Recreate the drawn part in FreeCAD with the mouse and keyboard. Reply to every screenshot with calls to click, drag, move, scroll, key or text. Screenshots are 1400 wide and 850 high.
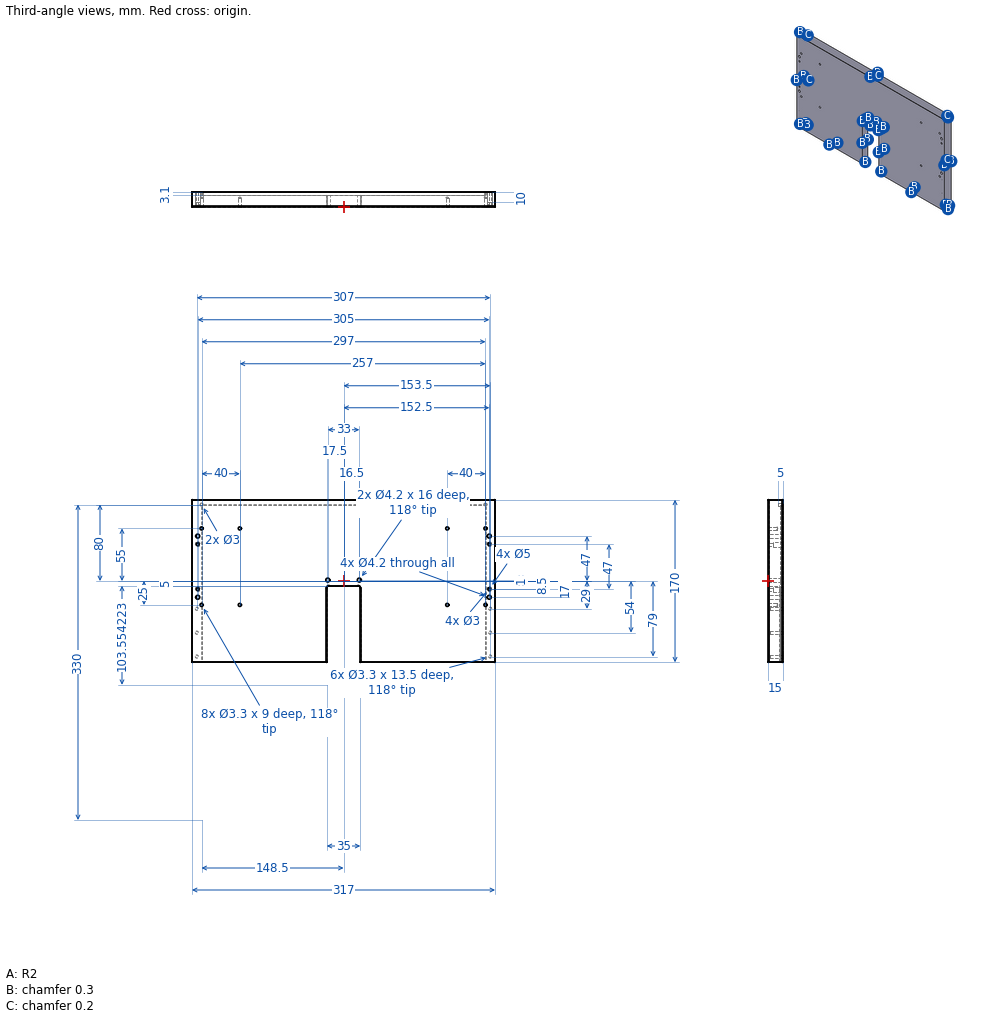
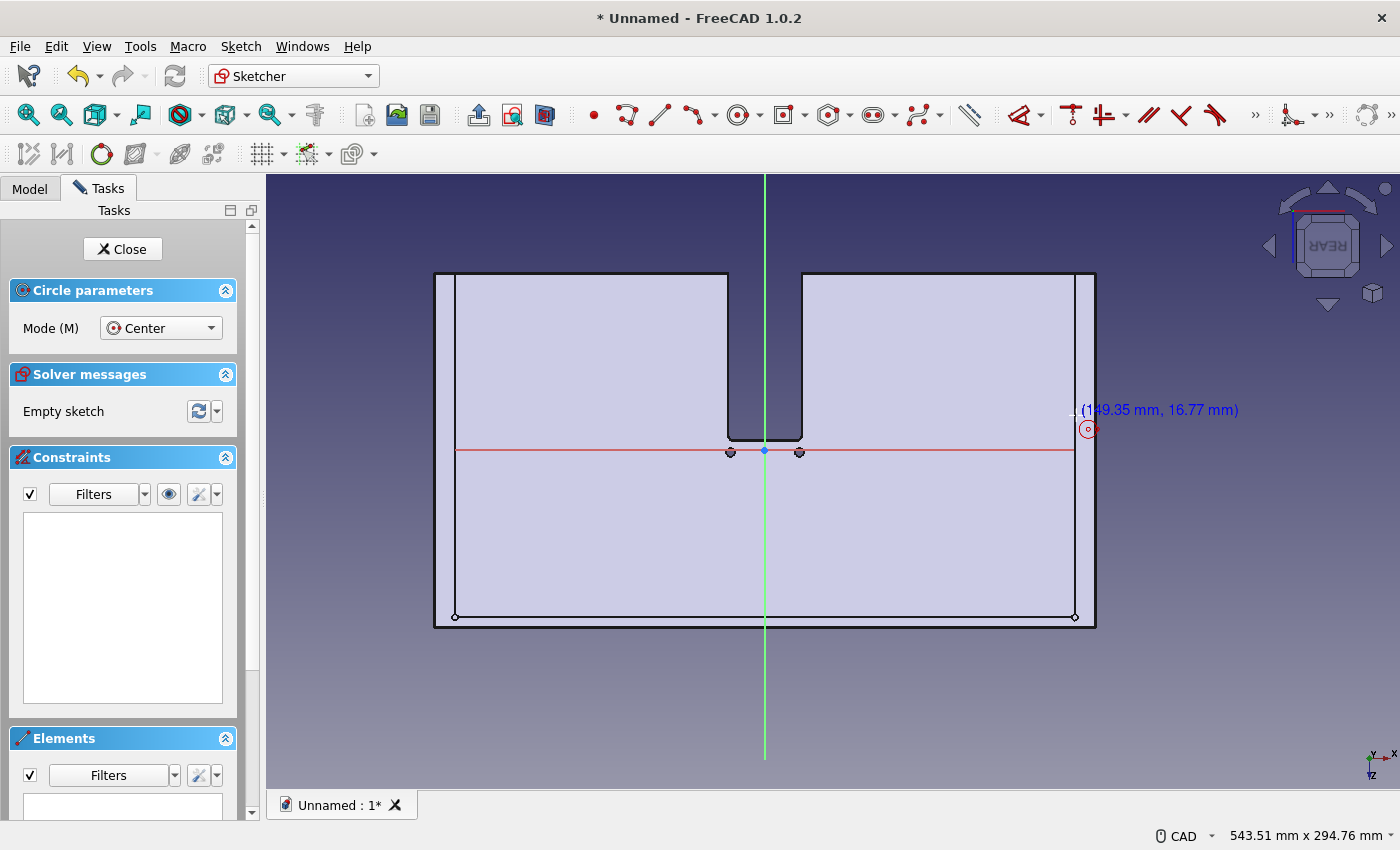
click(1083, 415)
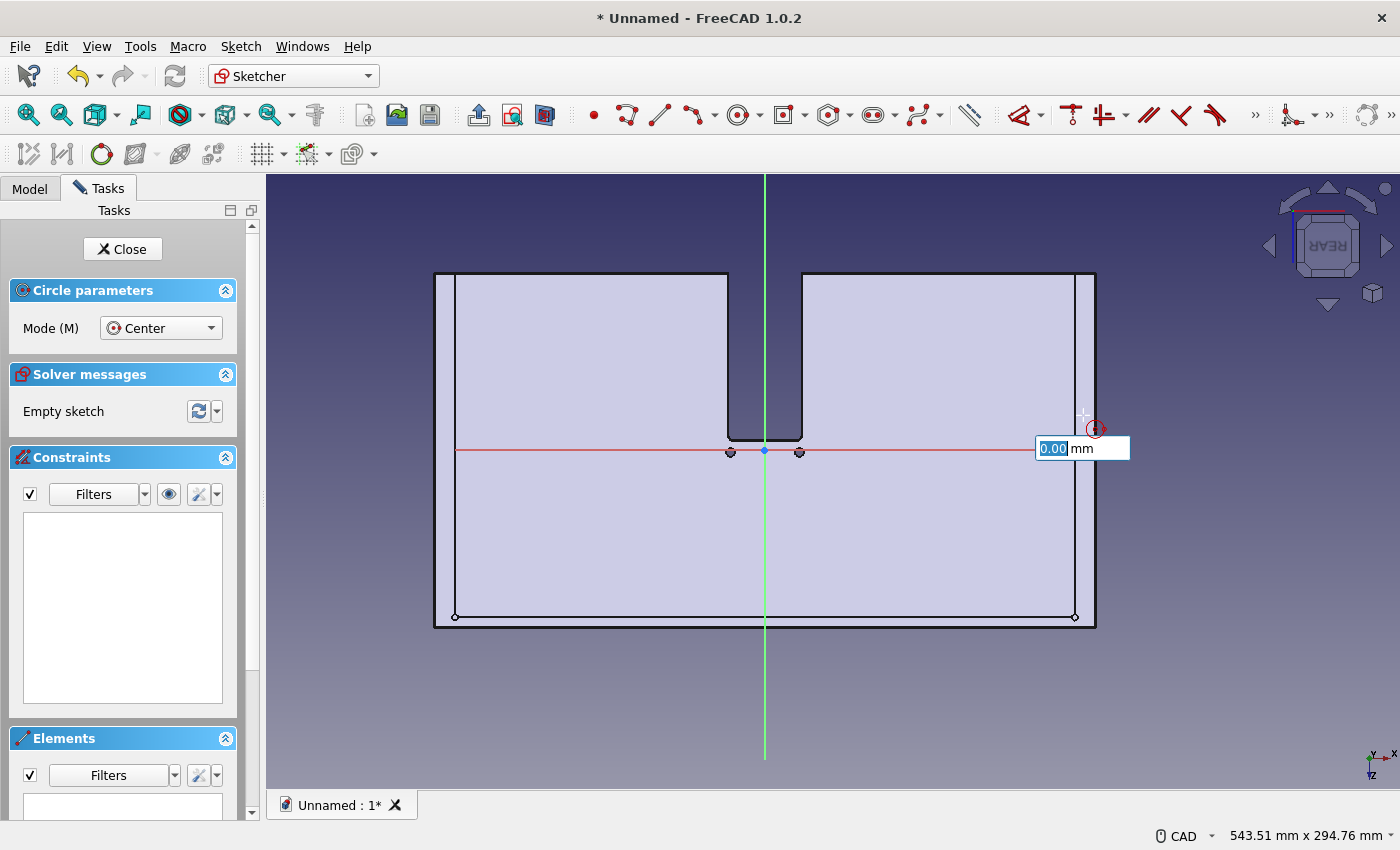
scroll(1086, 412, up, 7)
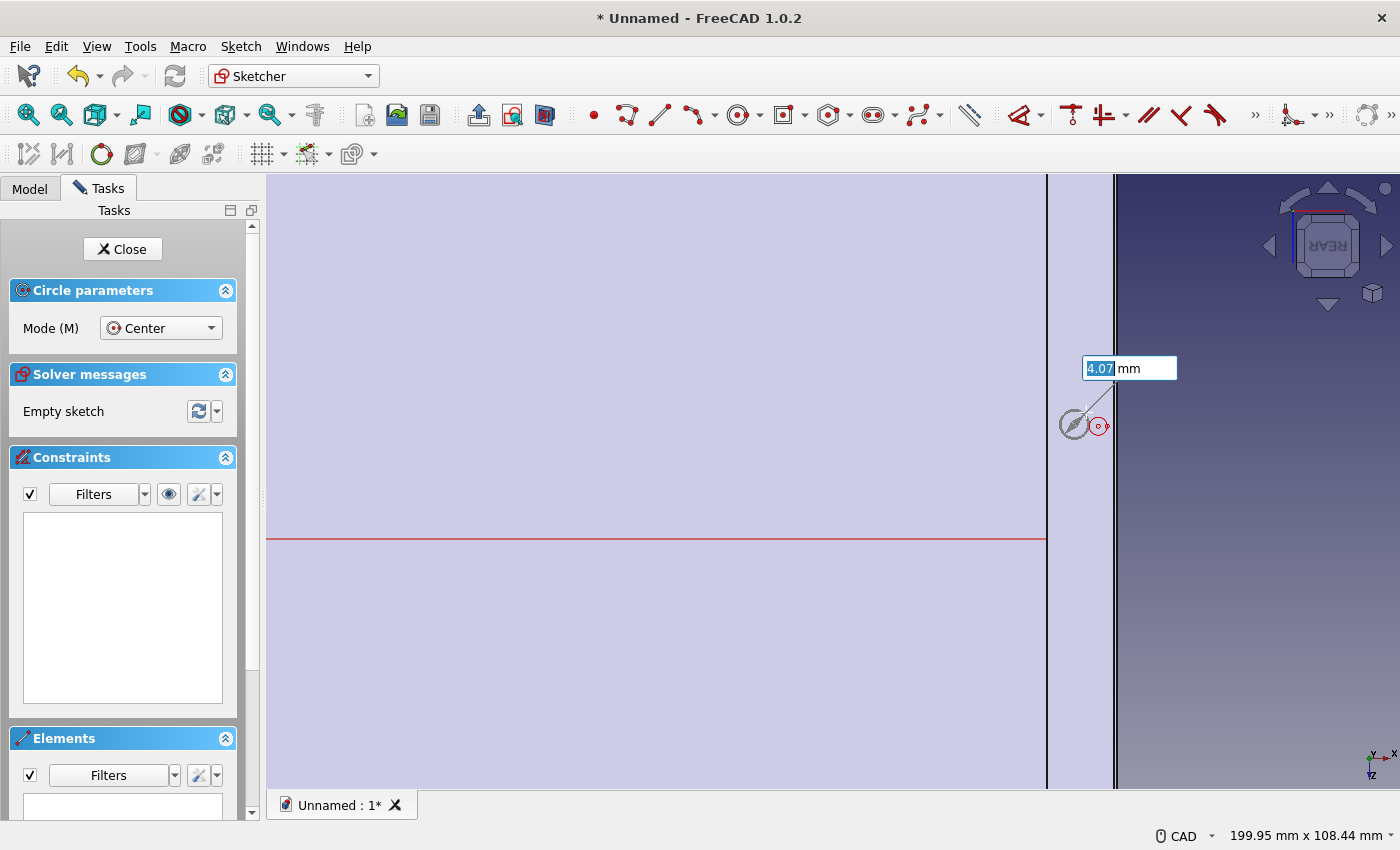
click(1085, 410)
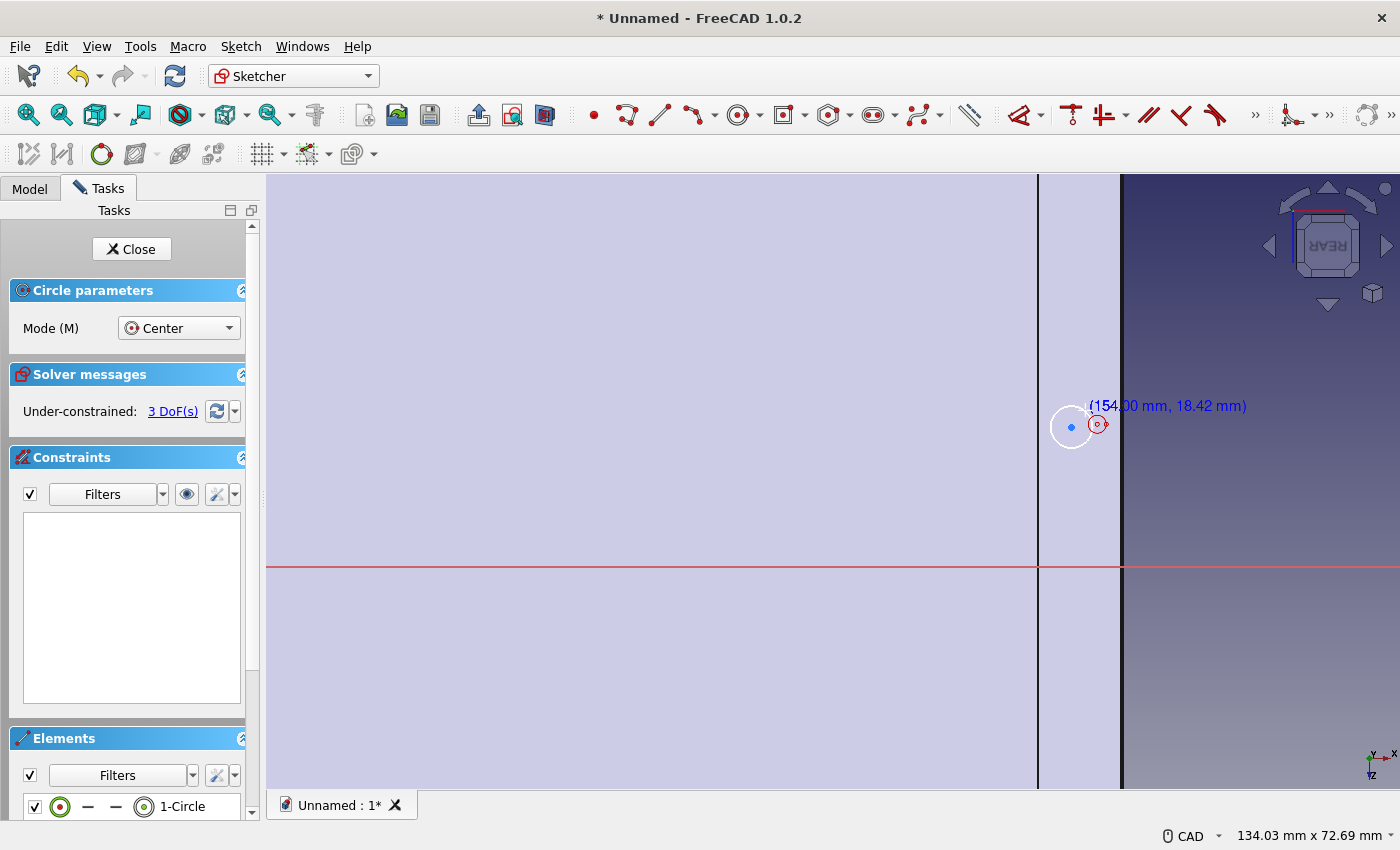
scroll(1086, 412, down, 7)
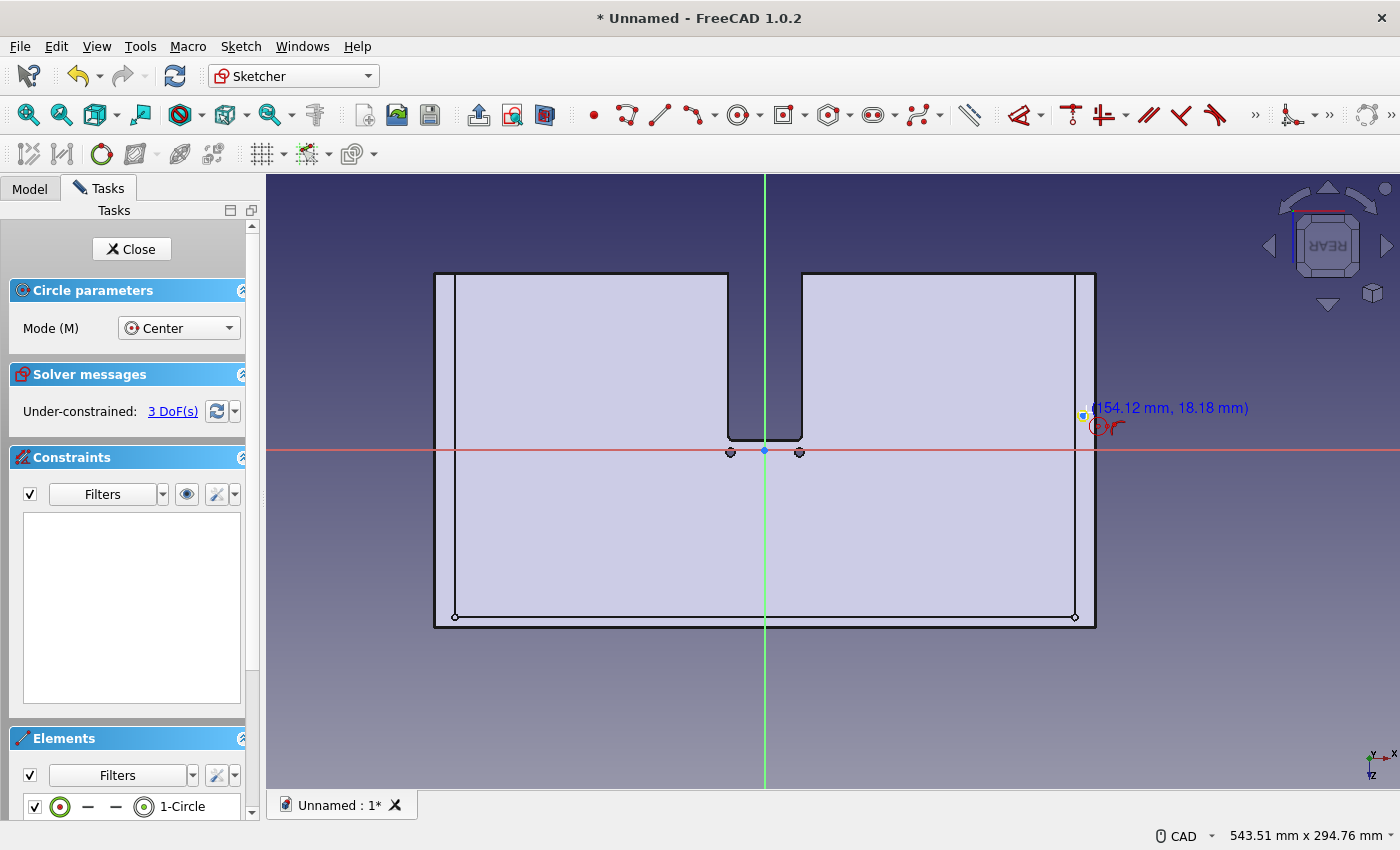
scroll(1083, 549, up, 9)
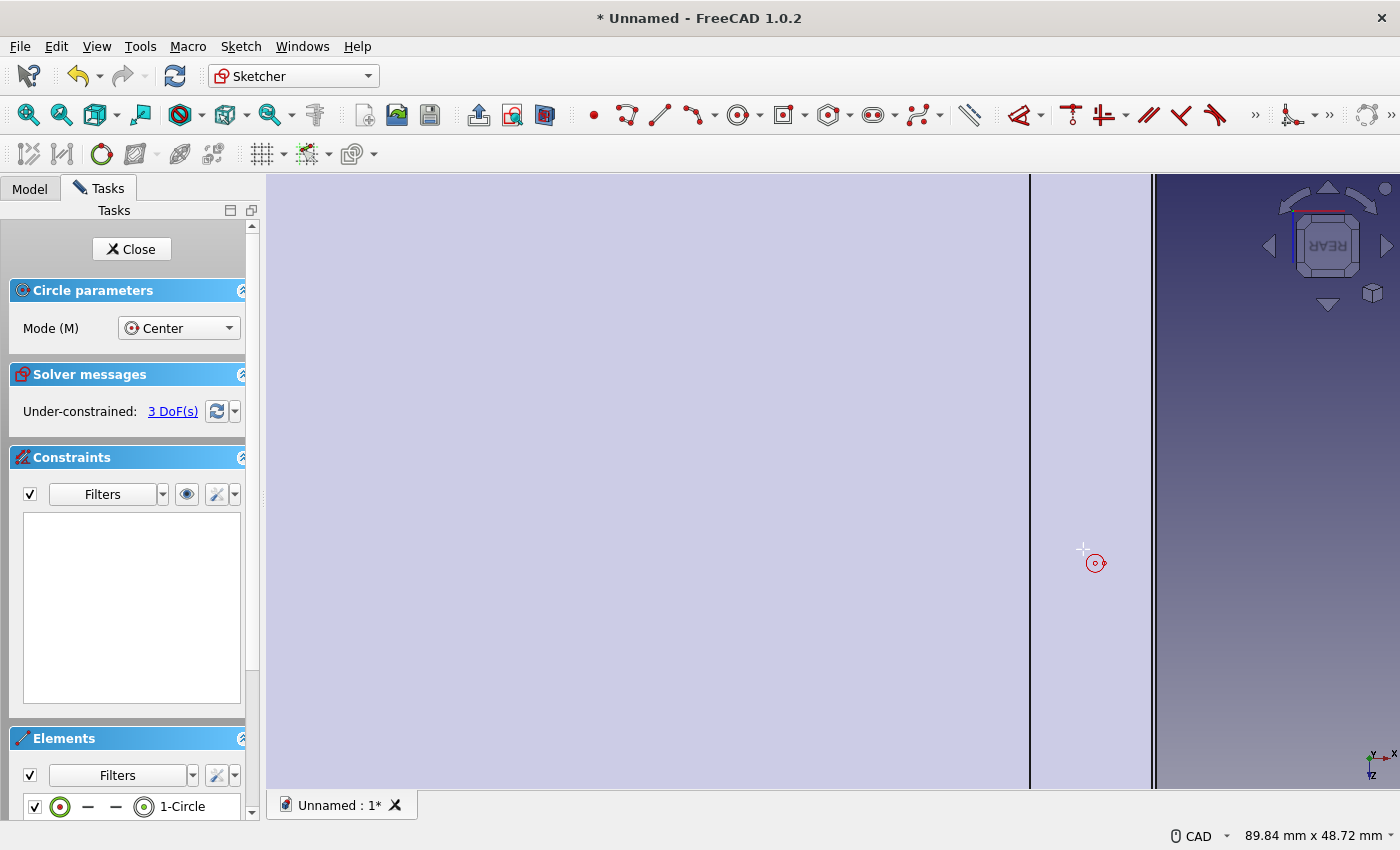
scroll(1083, 549, down, 9)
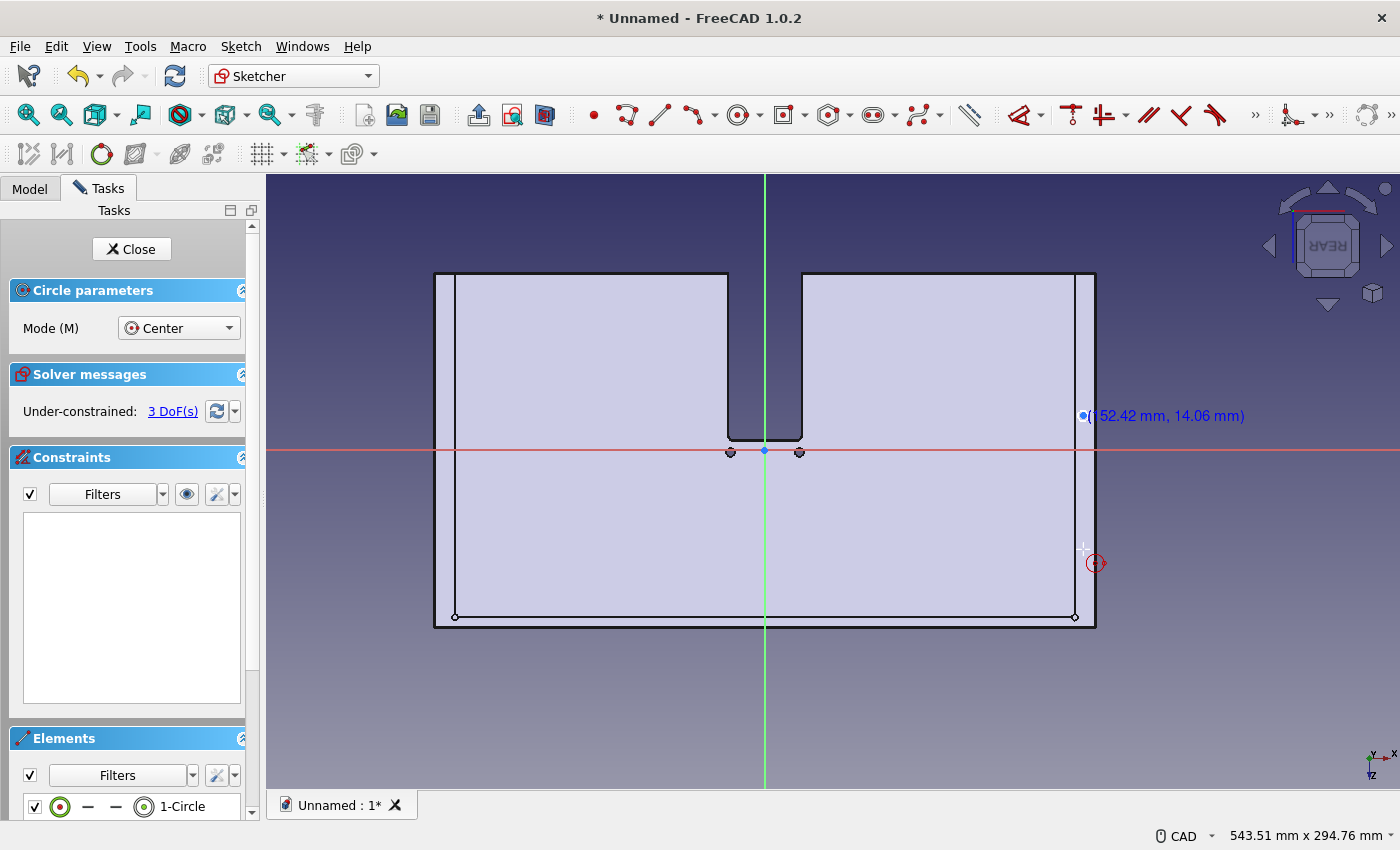
click(1083, 549)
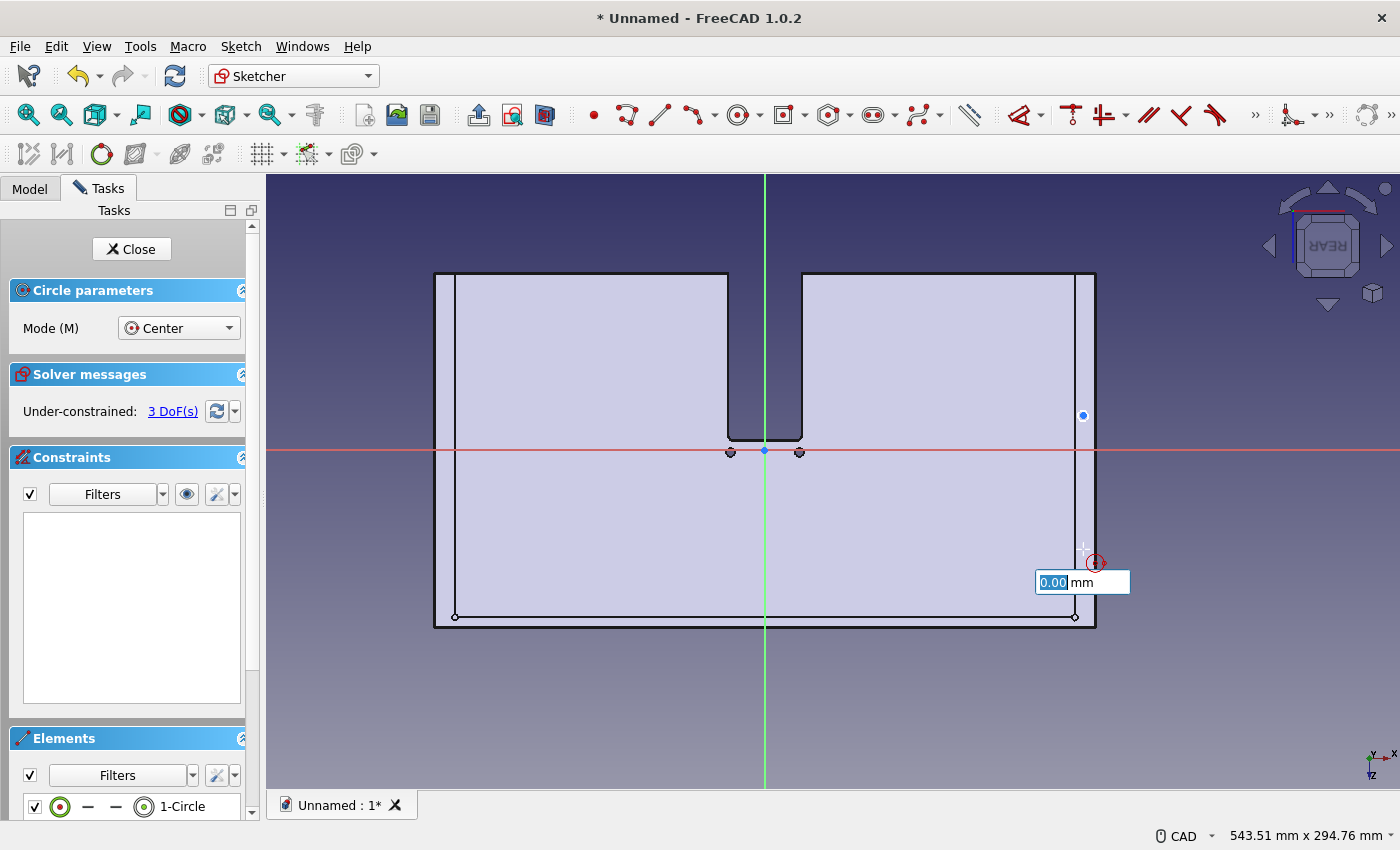
scroll(1086, 545, up, 7)